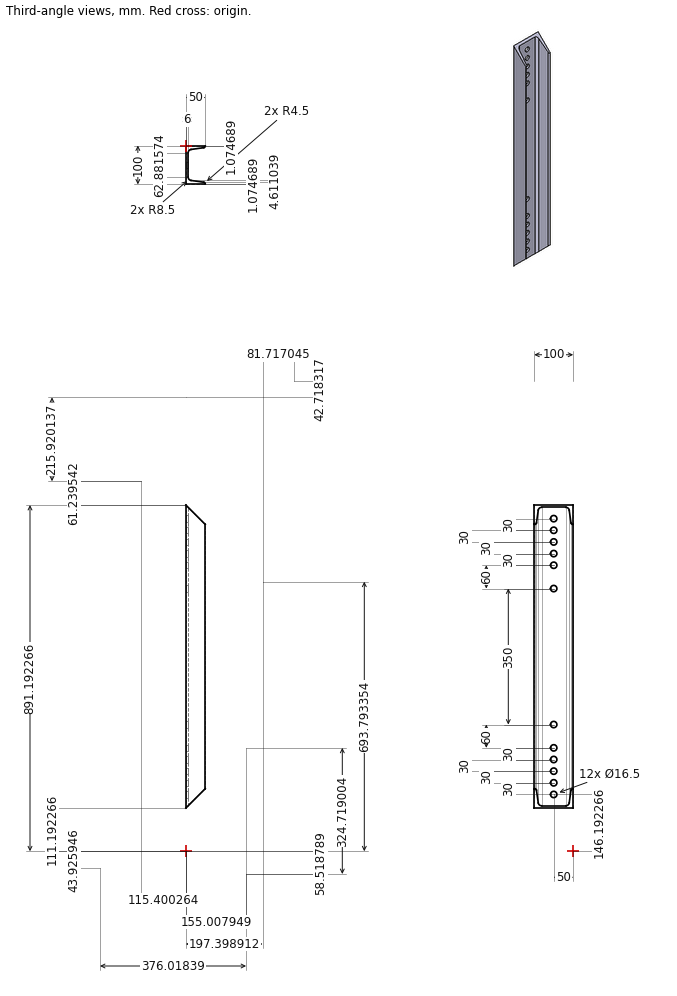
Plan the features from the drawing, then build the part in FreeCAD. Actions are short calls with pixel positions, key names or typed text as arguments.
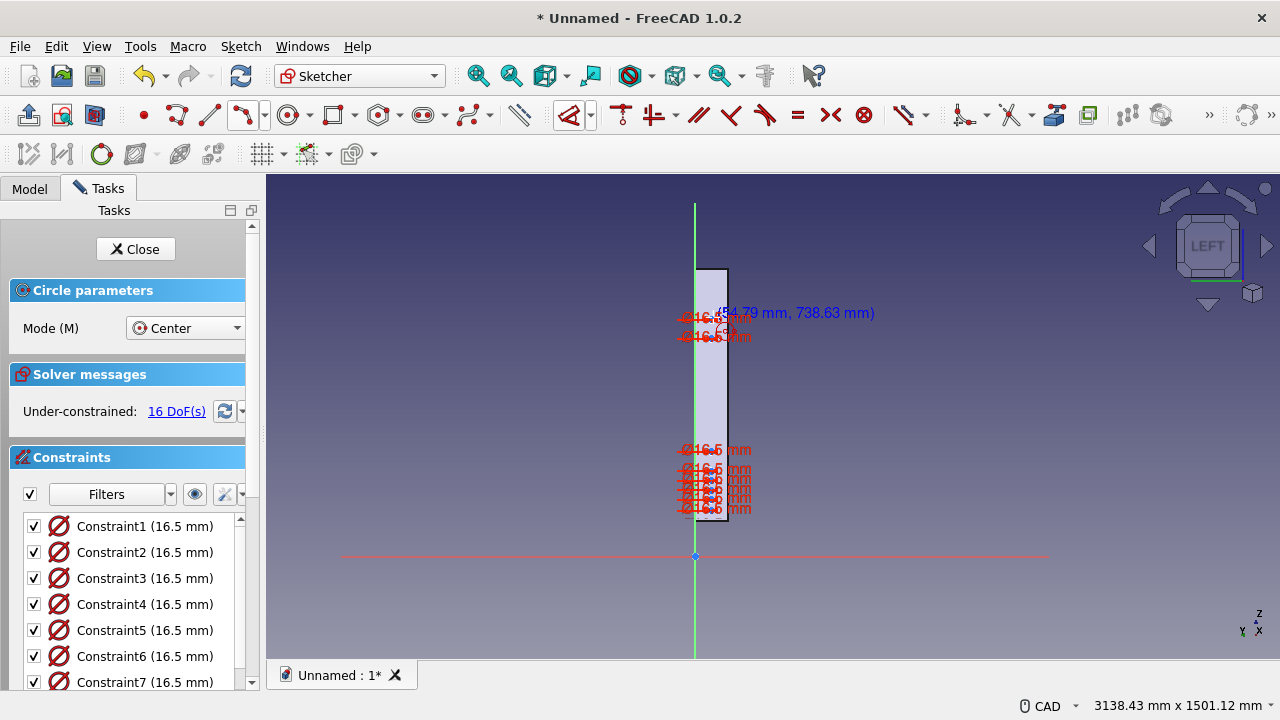
scroll(711, 309, up, 11)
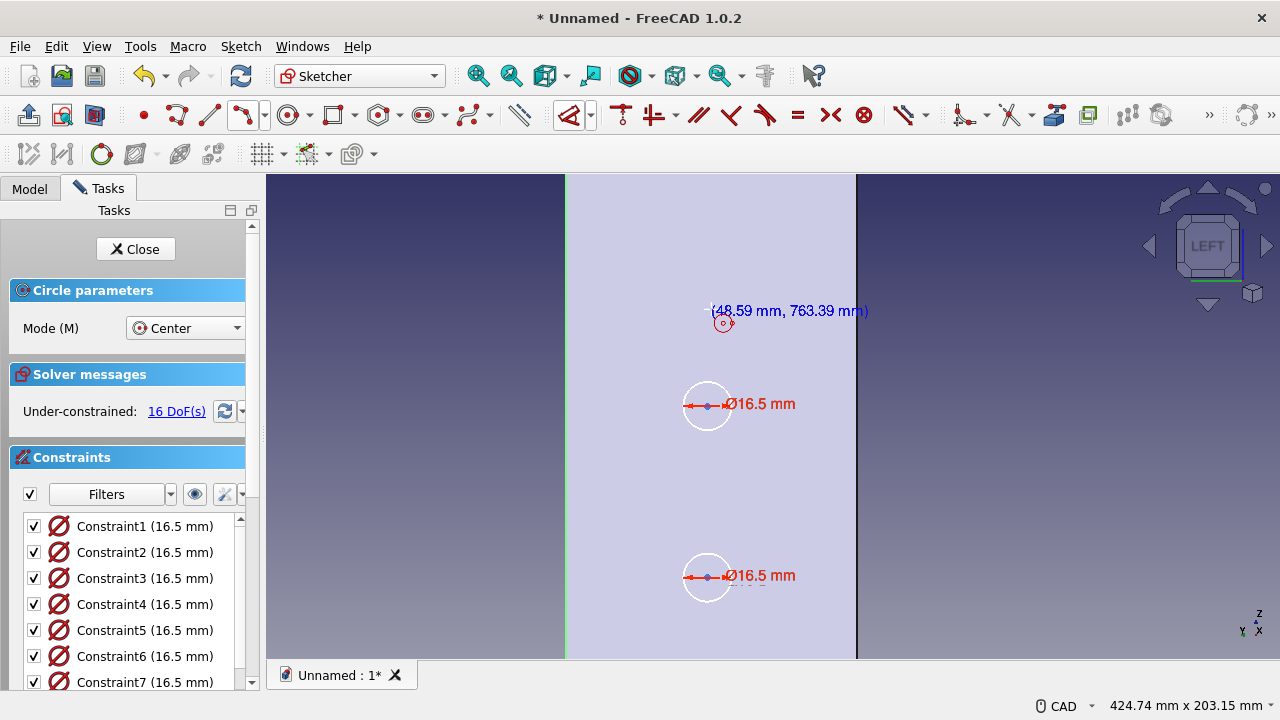
scroll(711, 309, down, 11)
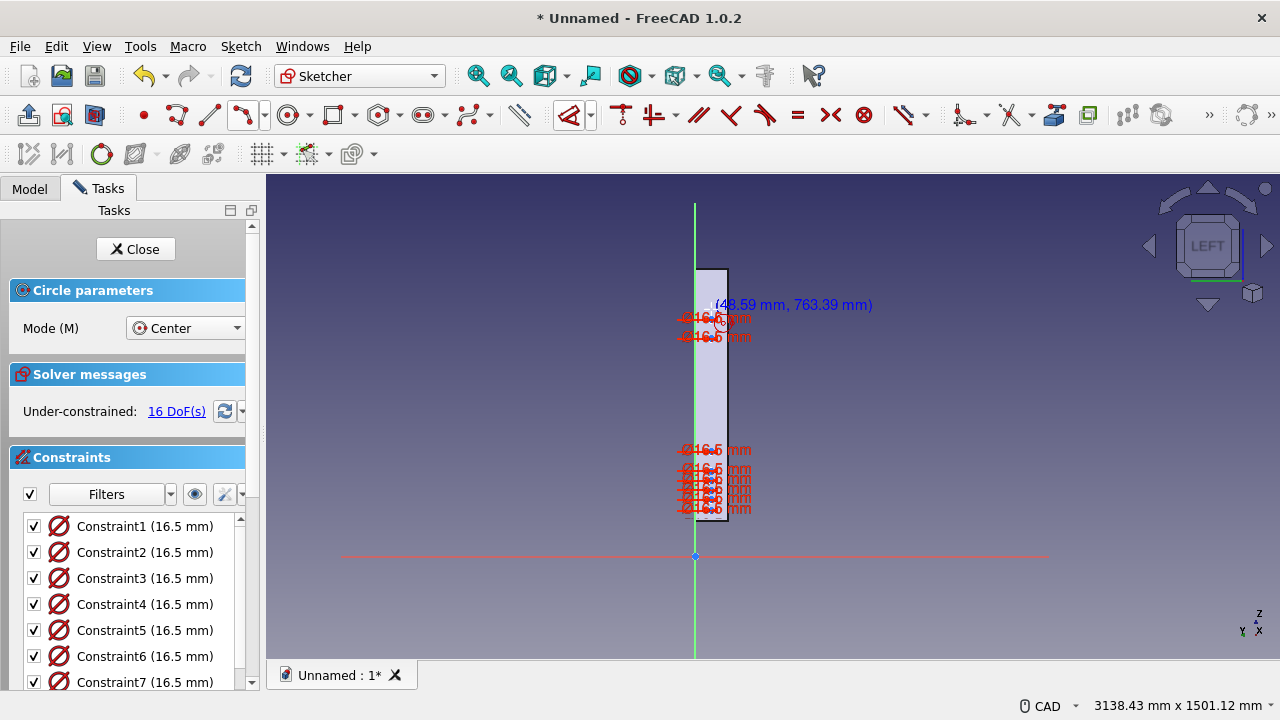
scroll(711, 309, up, 5)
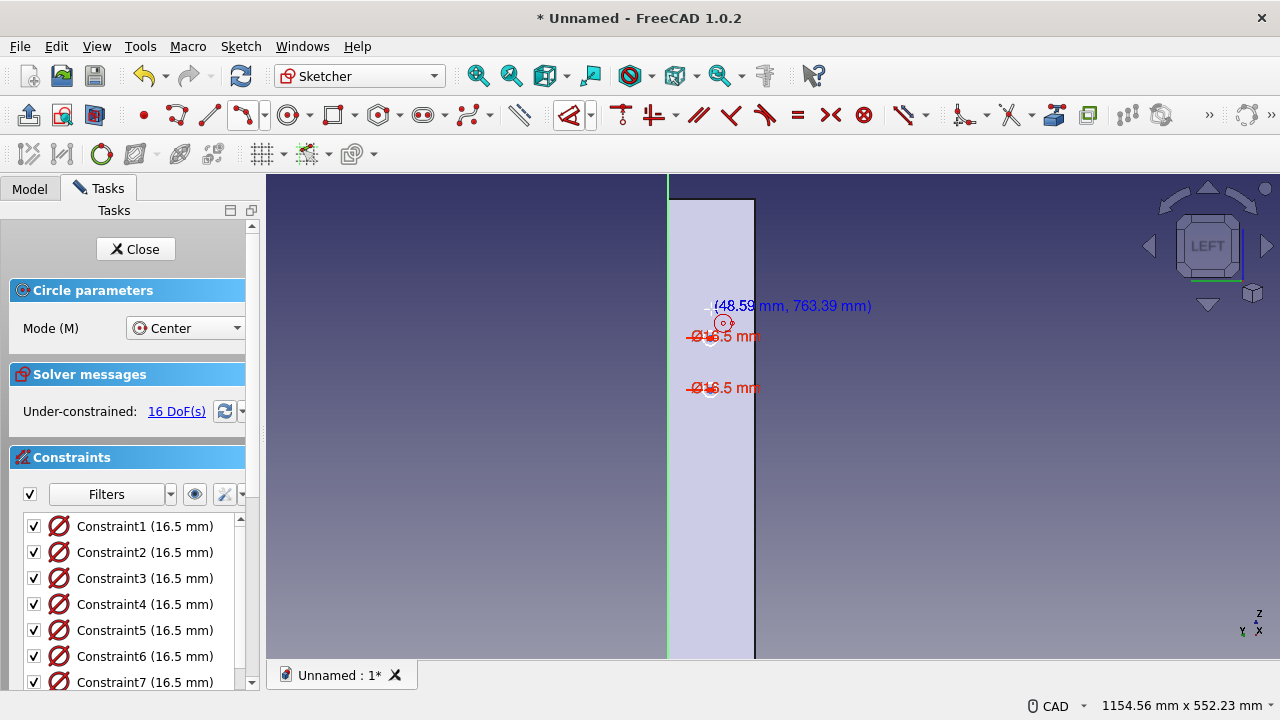
click(711, 309)
move(717, 304)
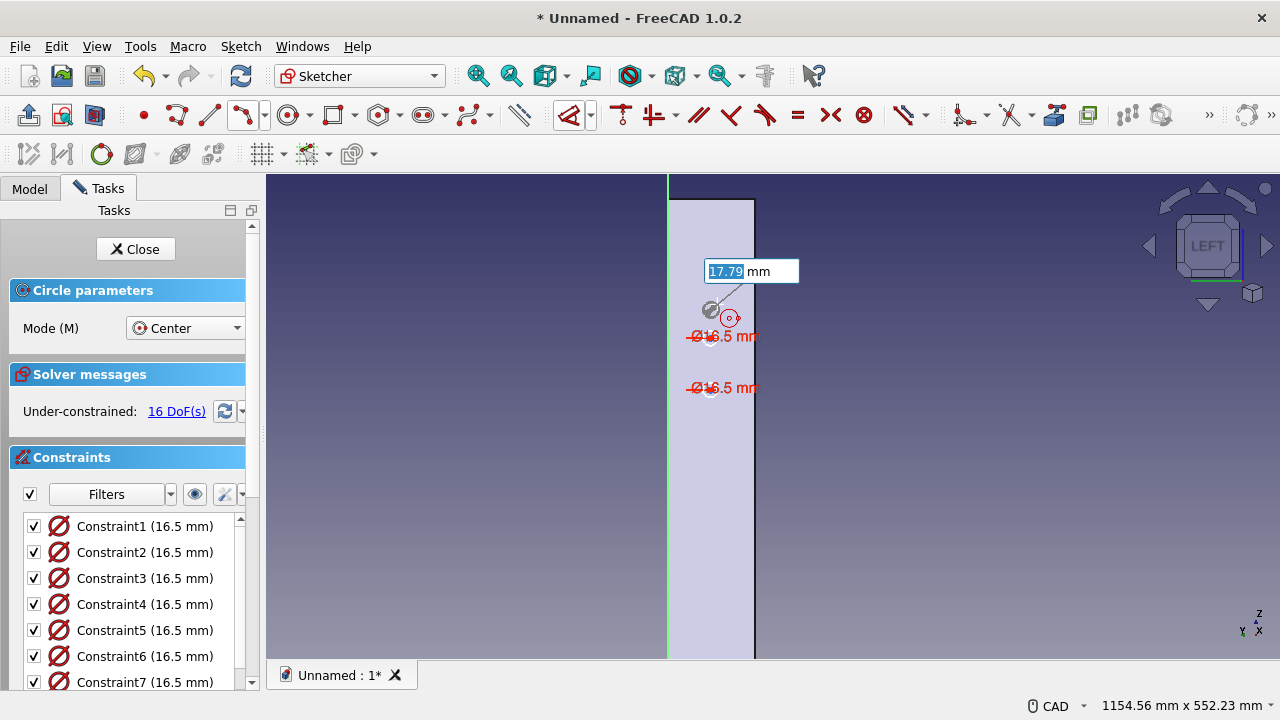
text(16.5)
key(Return)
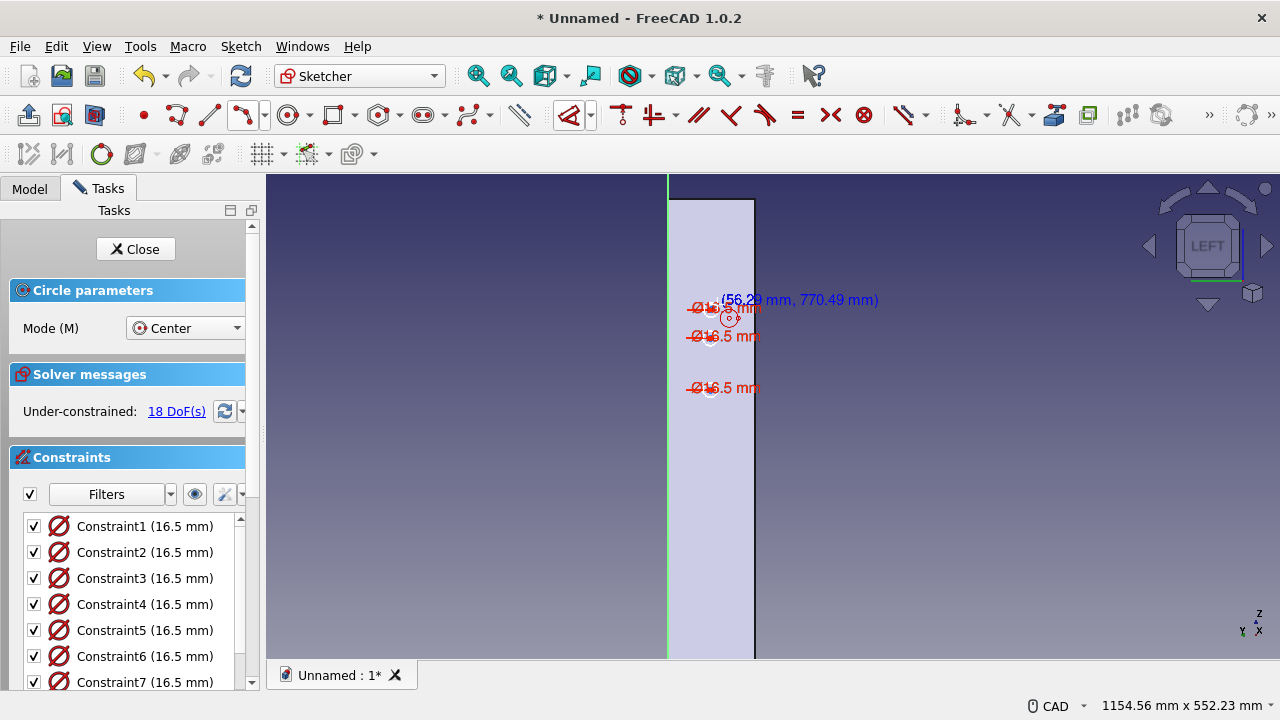
scroll(711, 282, up, 6)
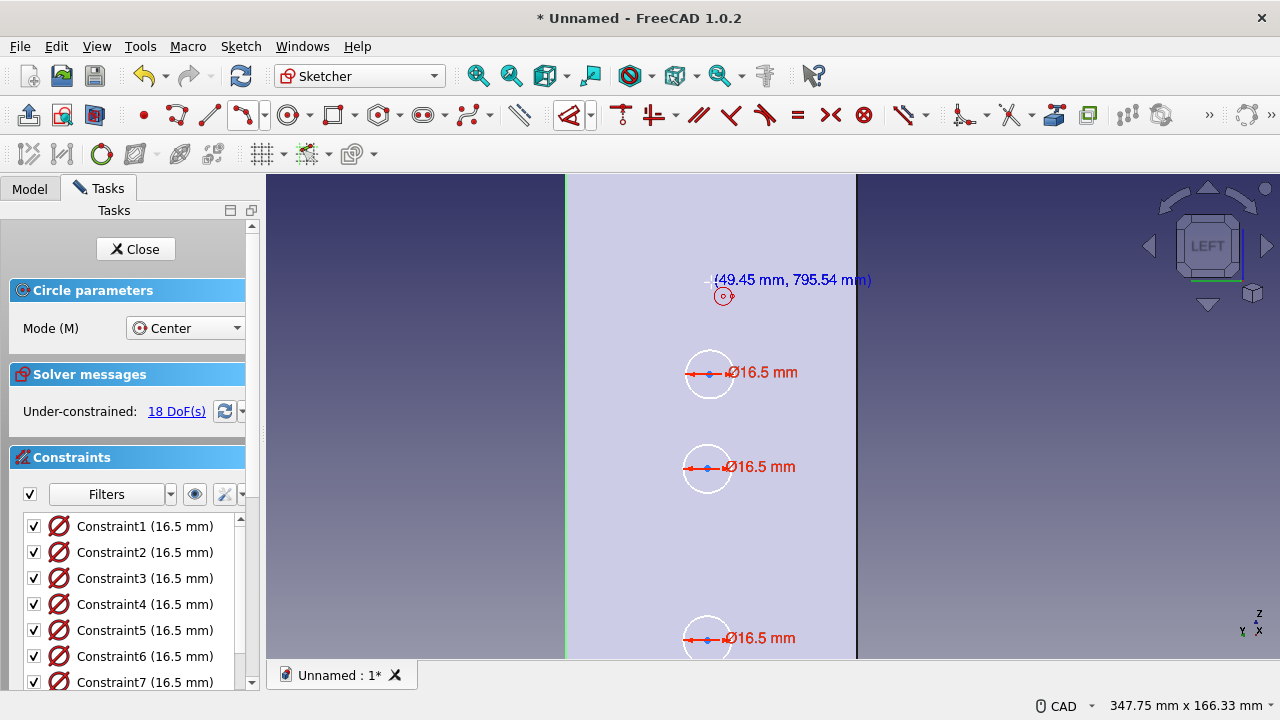
scroll(711, 301, down, 11)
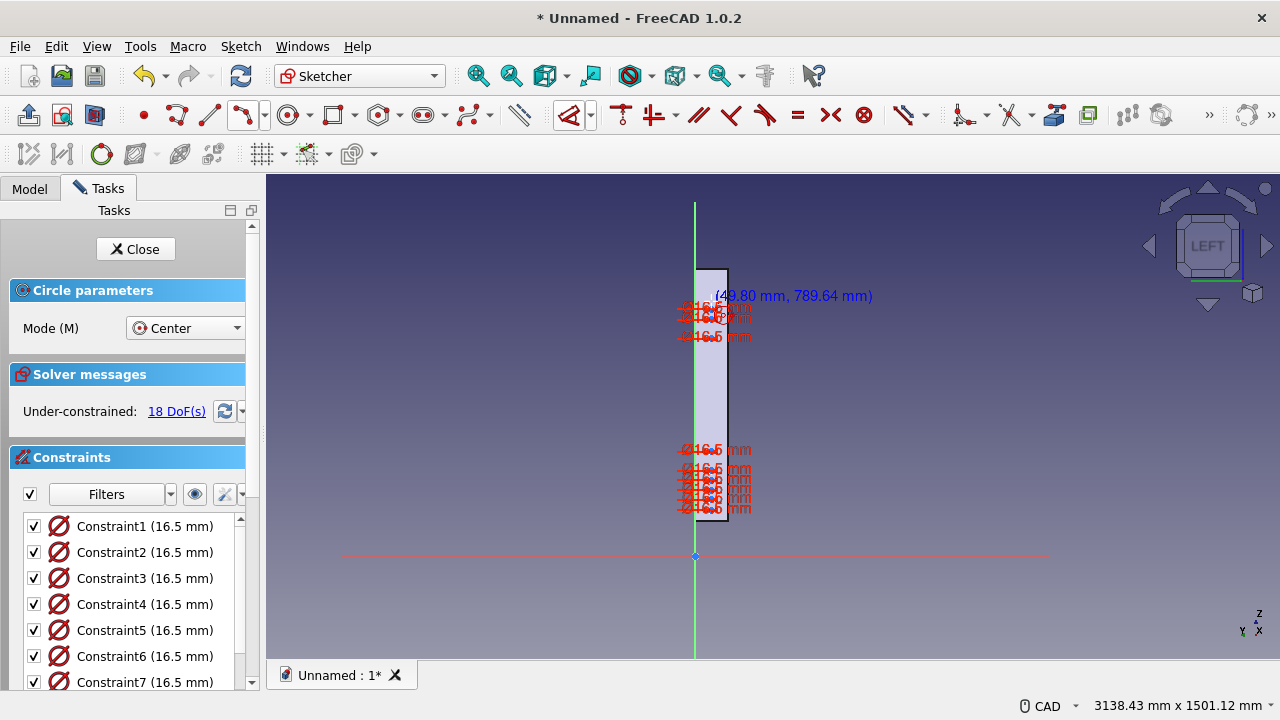
scroll(711, 299, up, 5)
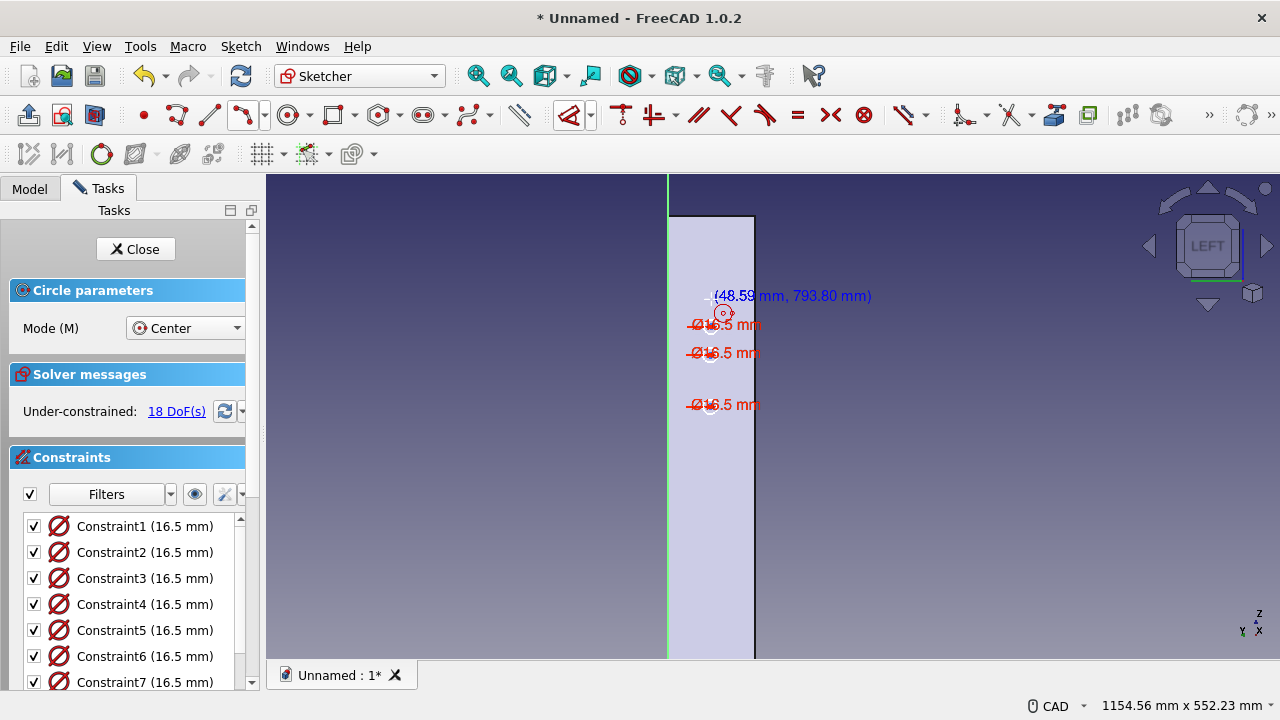
click(711, 299)
move(717, 294)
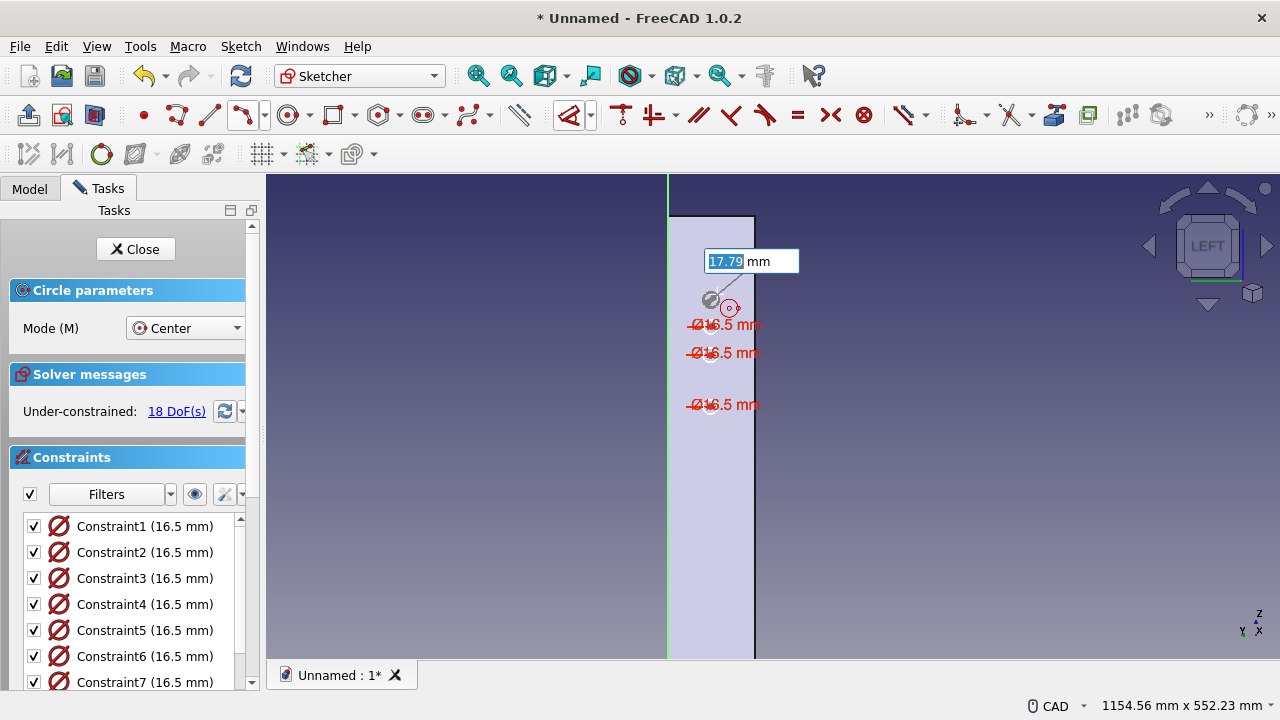
text(16.5)
key(Return)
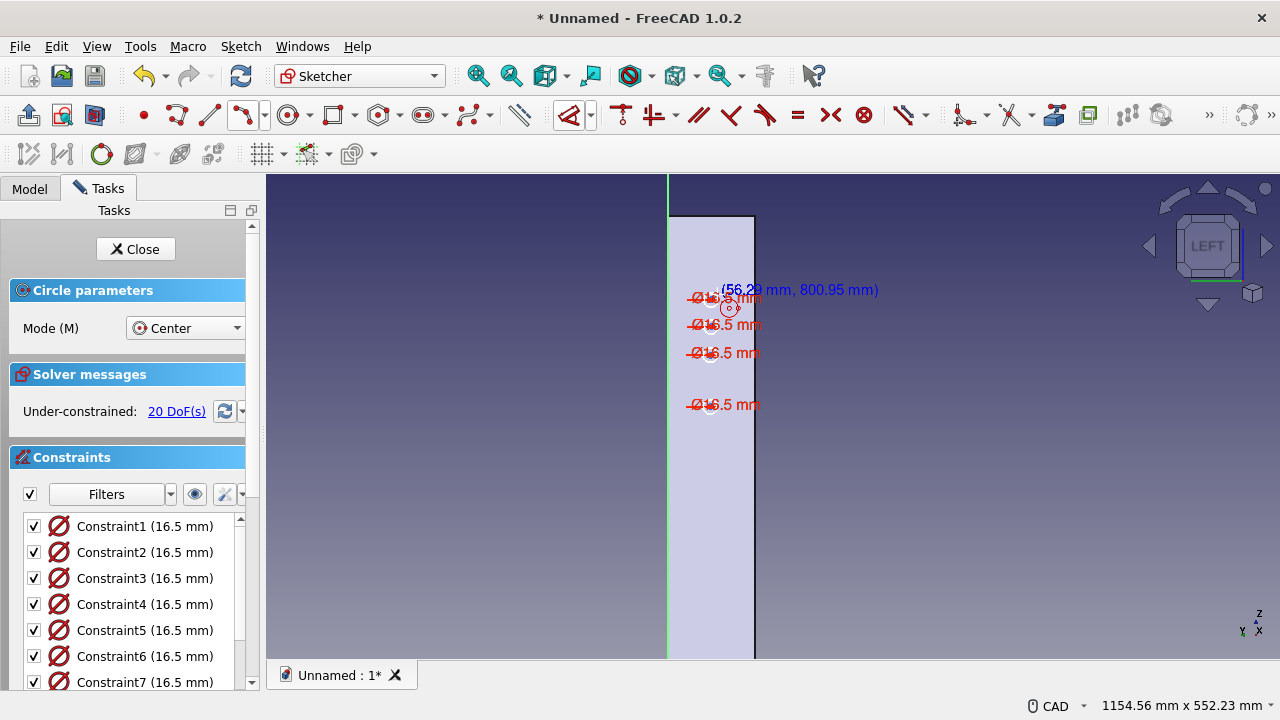
scroll(711, 273, up, 6)